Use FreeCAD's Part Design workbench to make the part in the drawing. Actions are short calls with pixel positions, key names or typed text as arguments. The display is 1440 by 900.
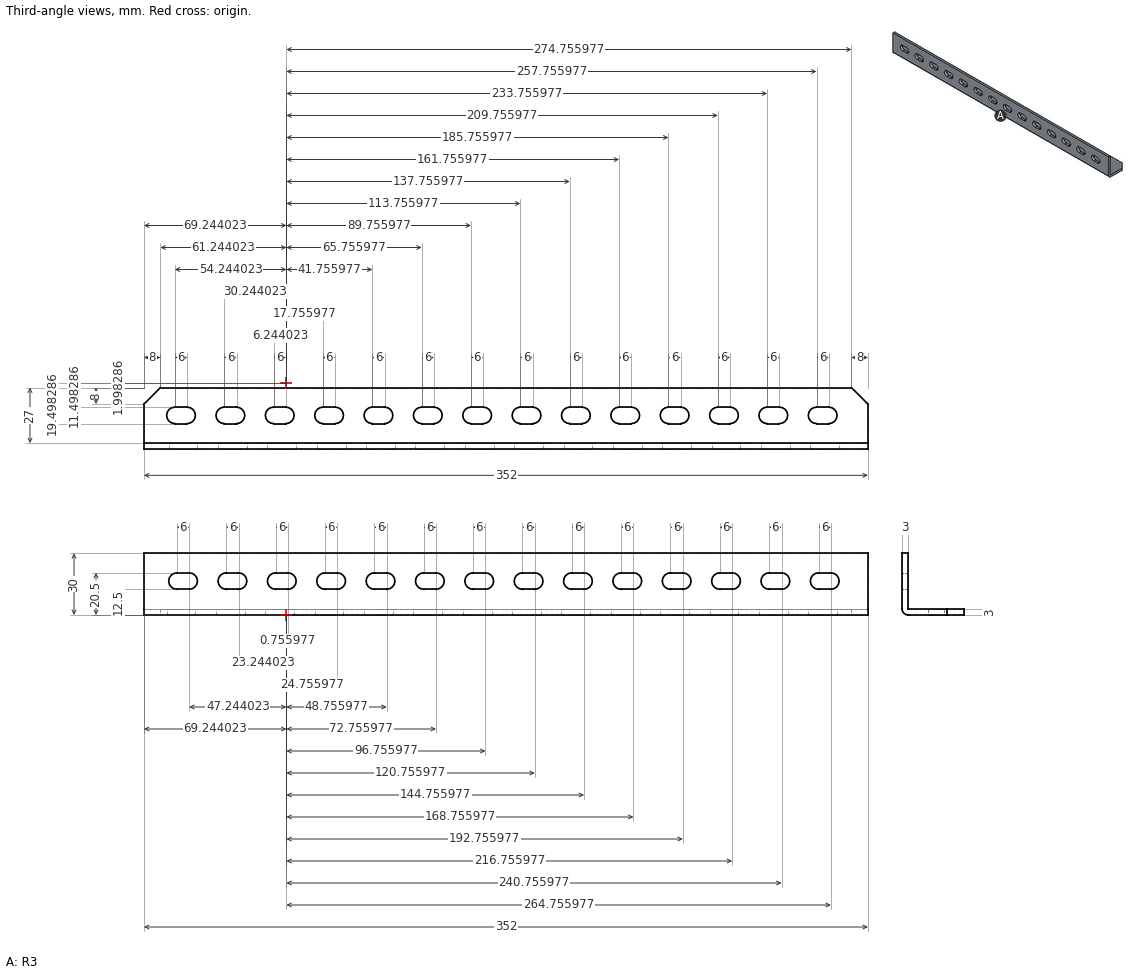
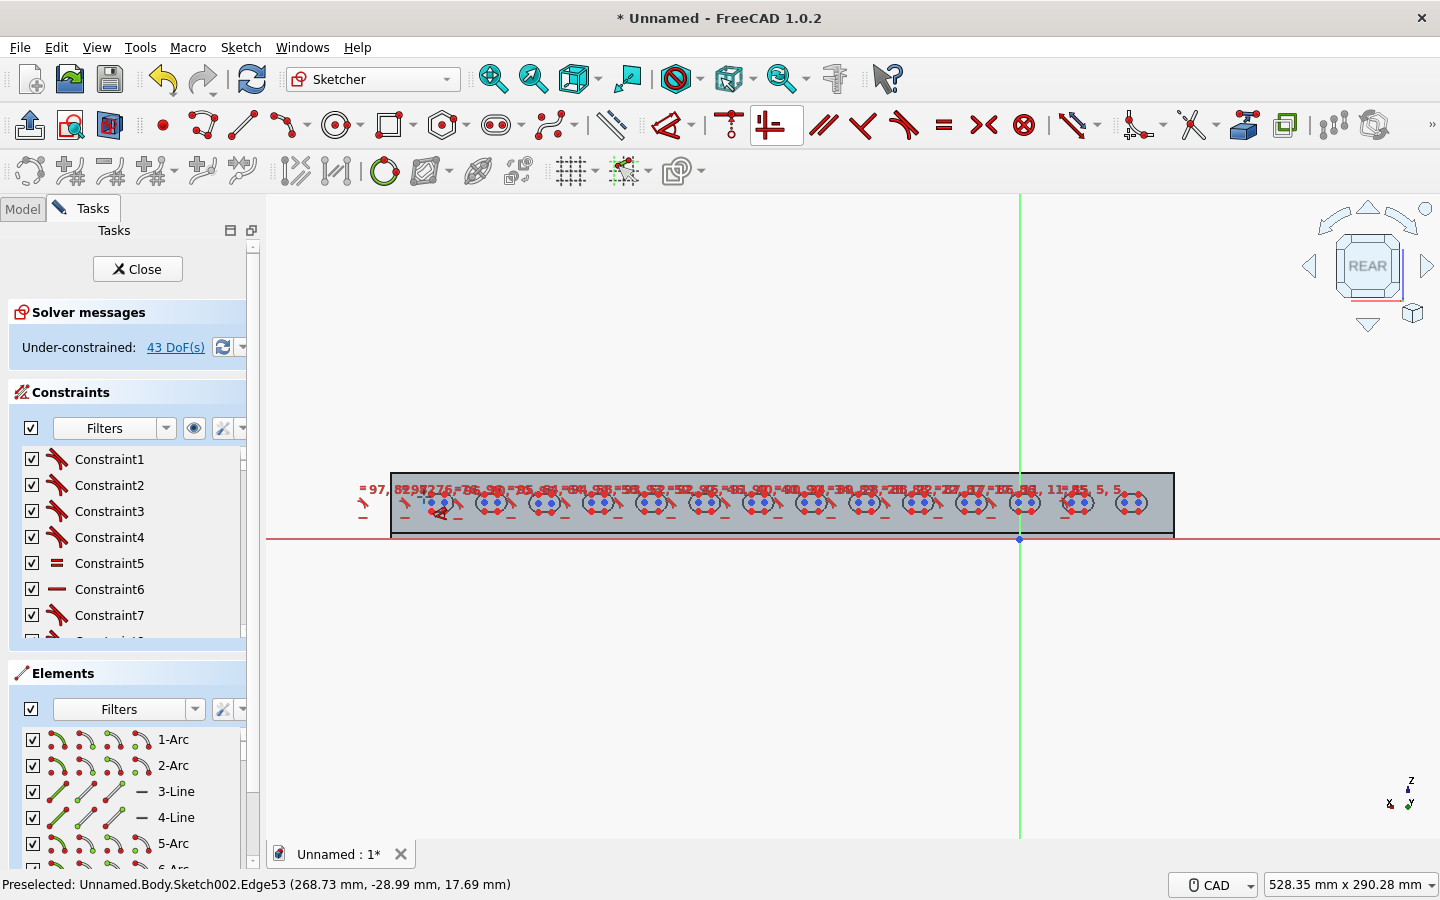
scroll(1130, 494, up, 6)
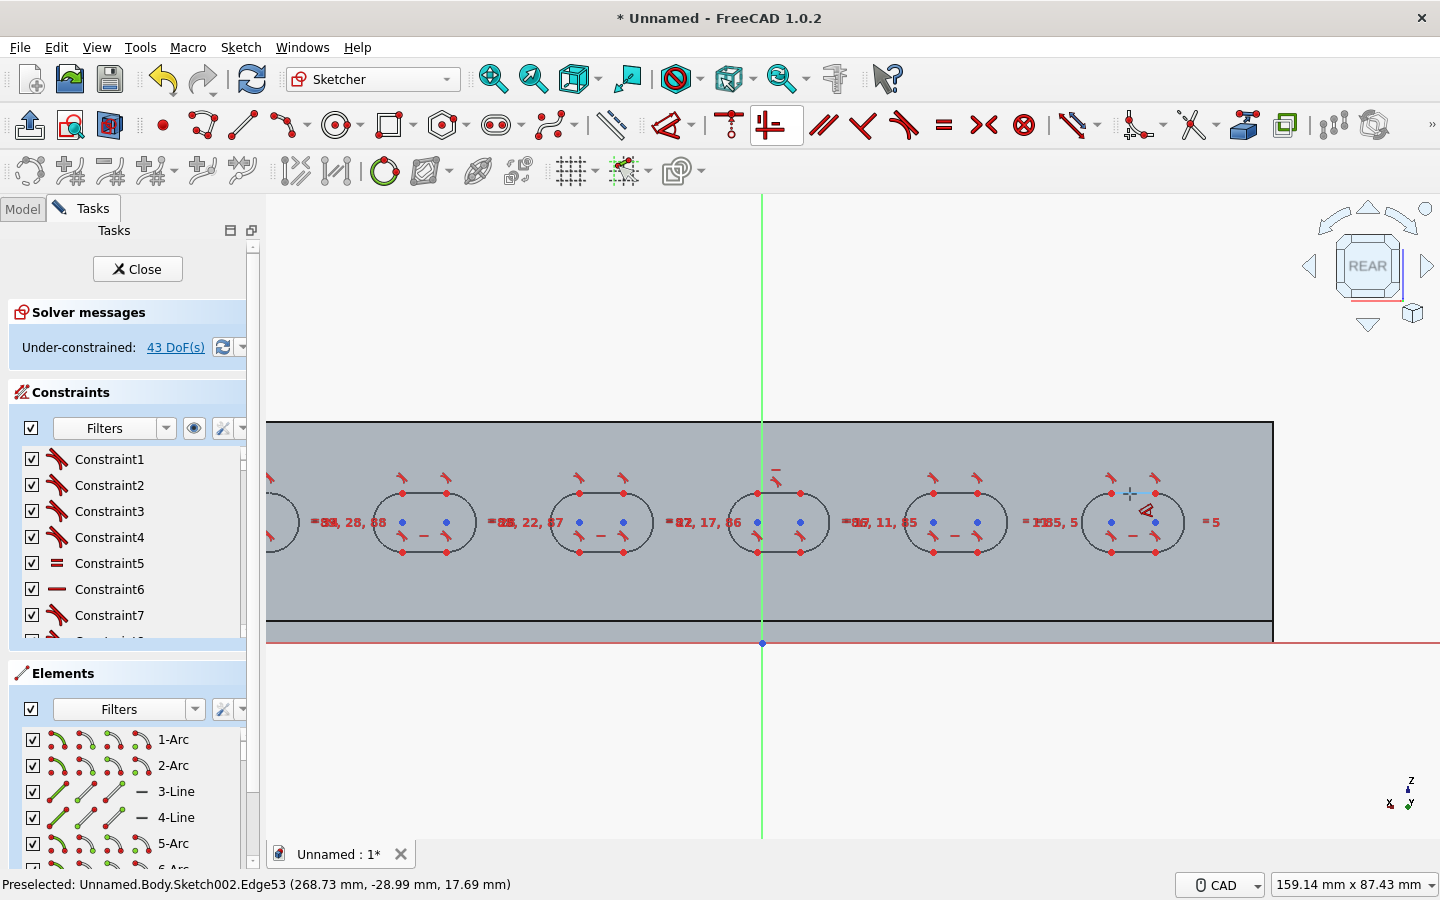
click(1129, 493)
click(1133, 459)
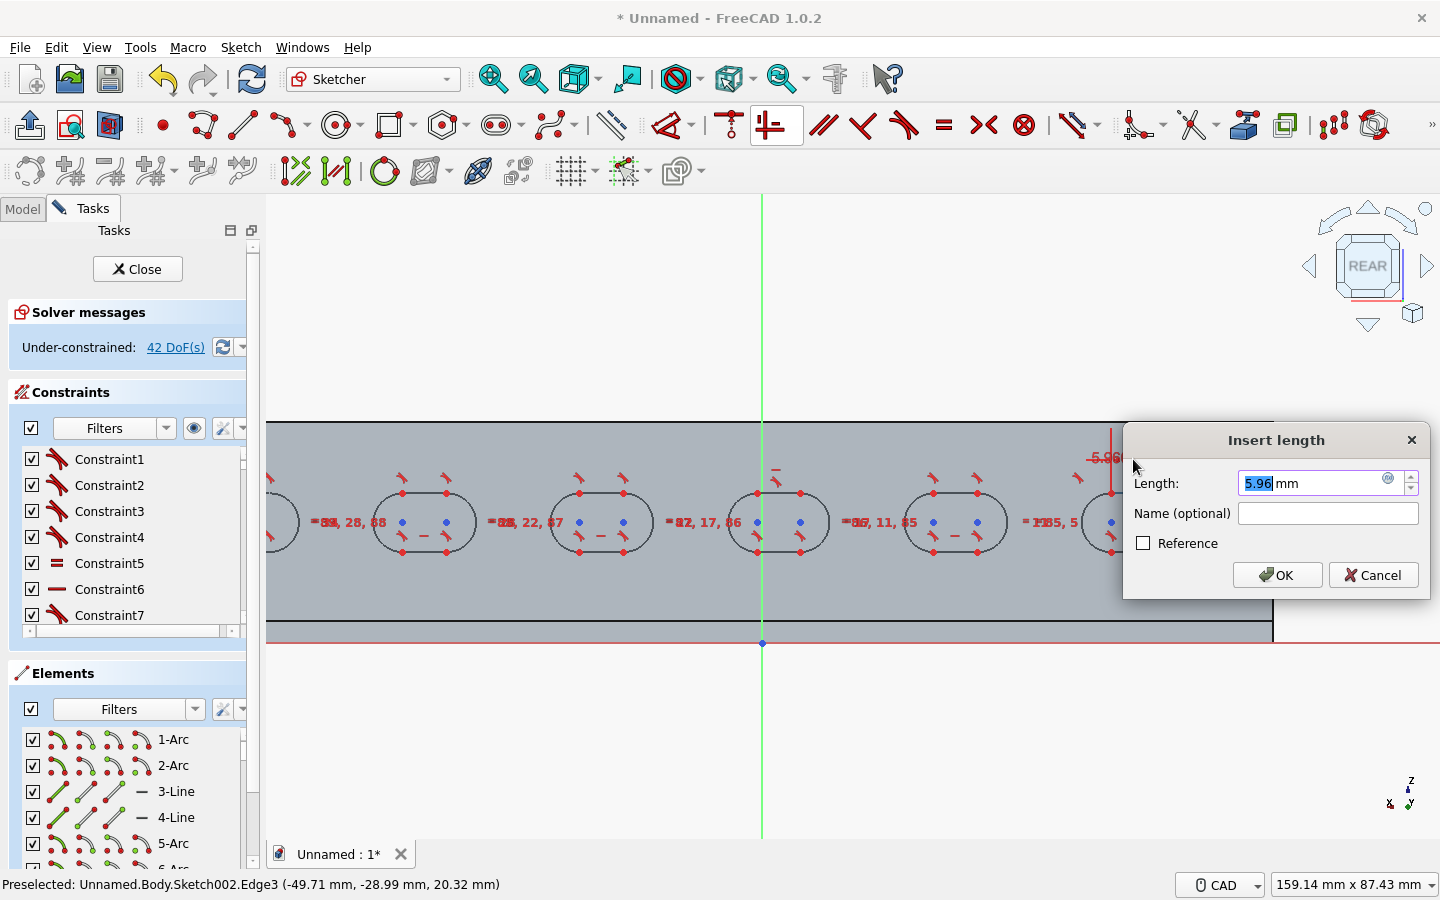
text(6)
key(Return)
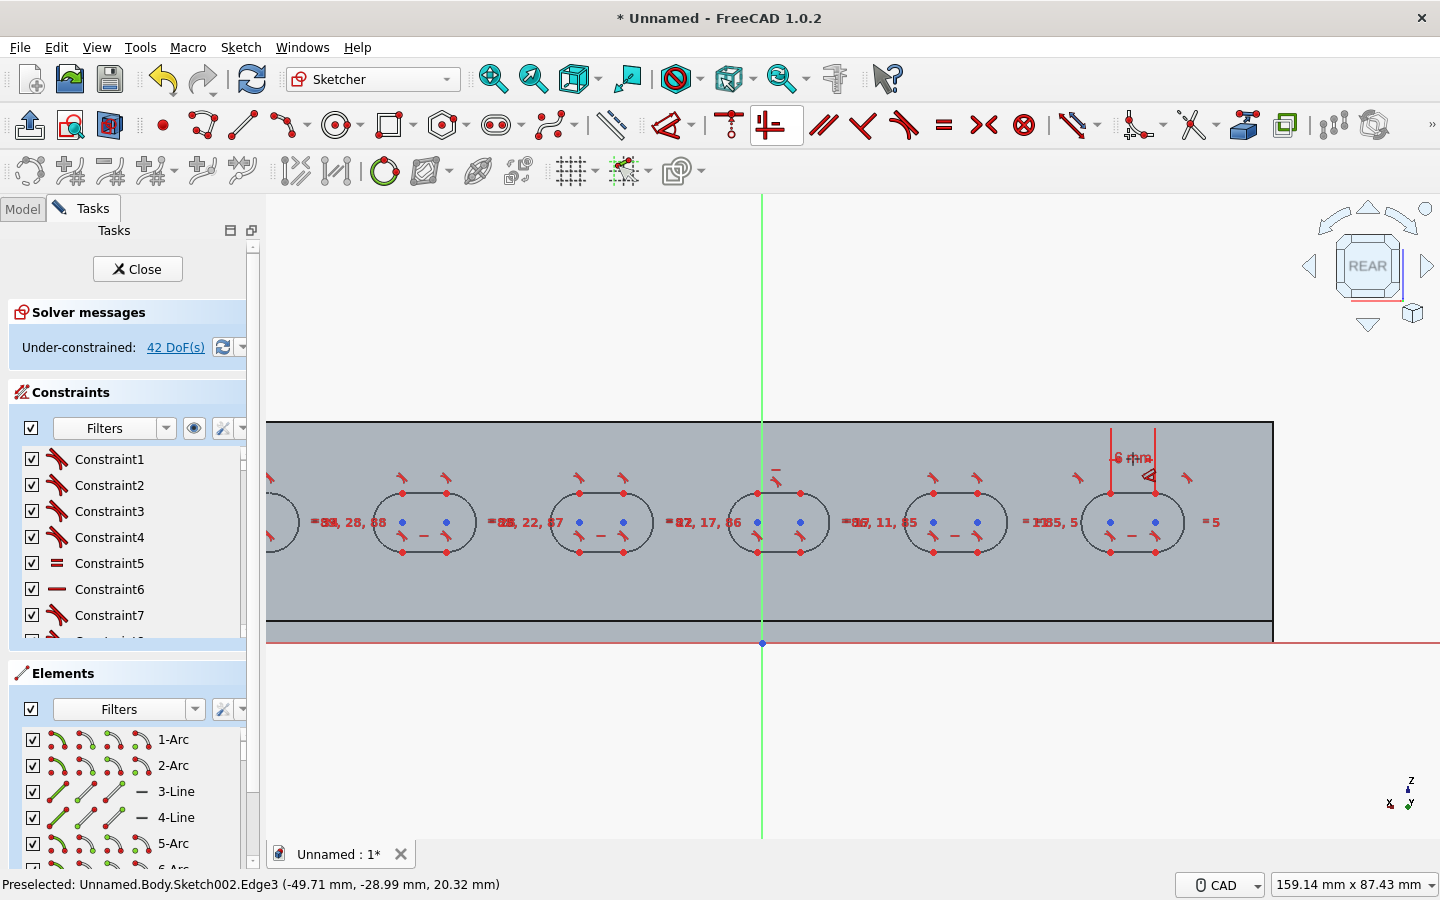
click(947, 493)
click(956, 459)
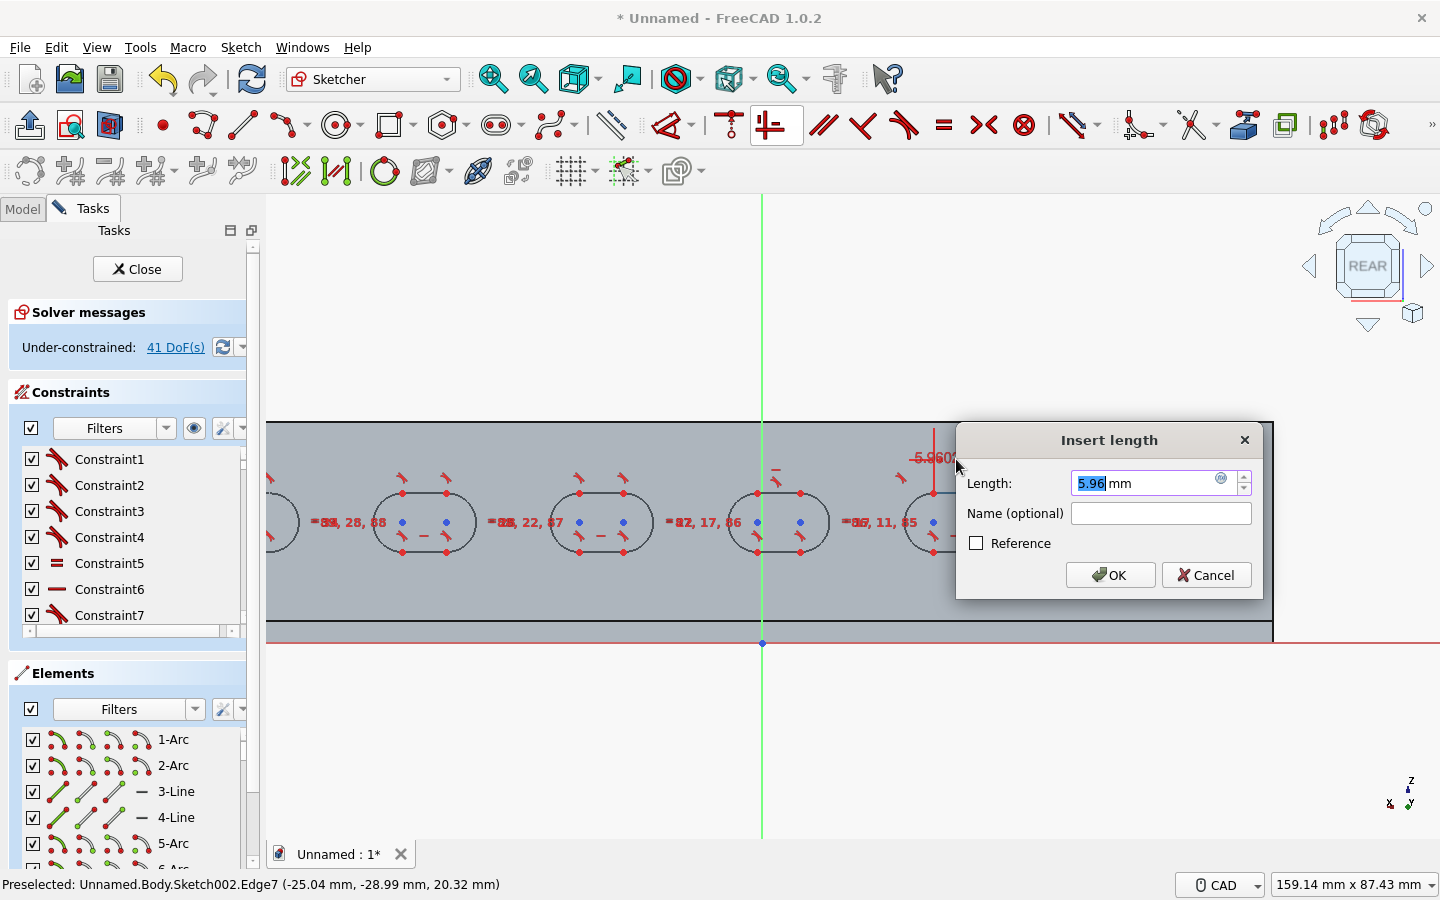
text(6)
key(Return)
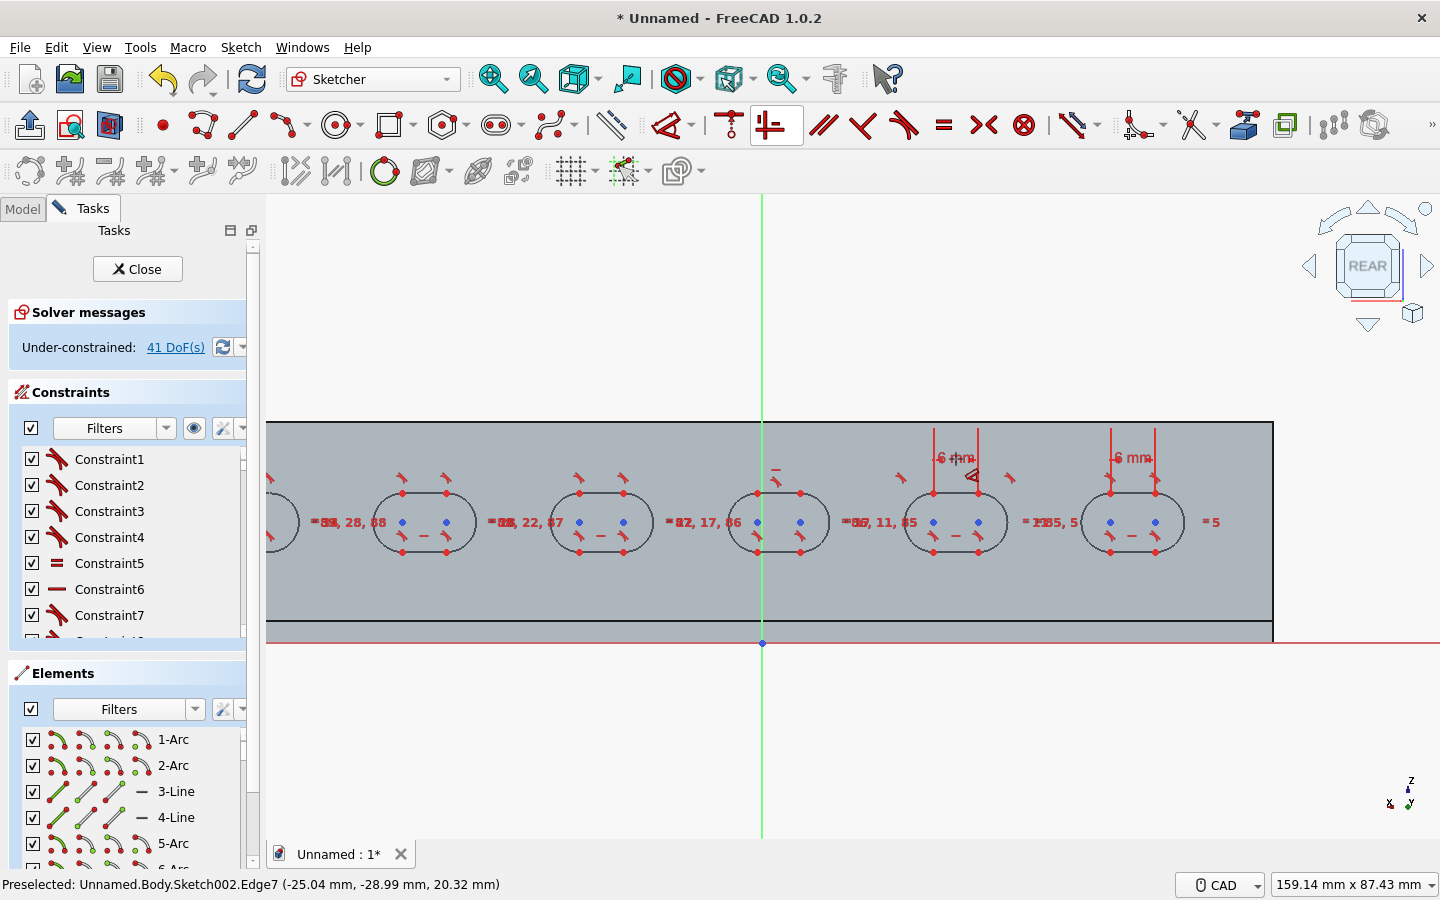
click(787, 493)
click(779, 459)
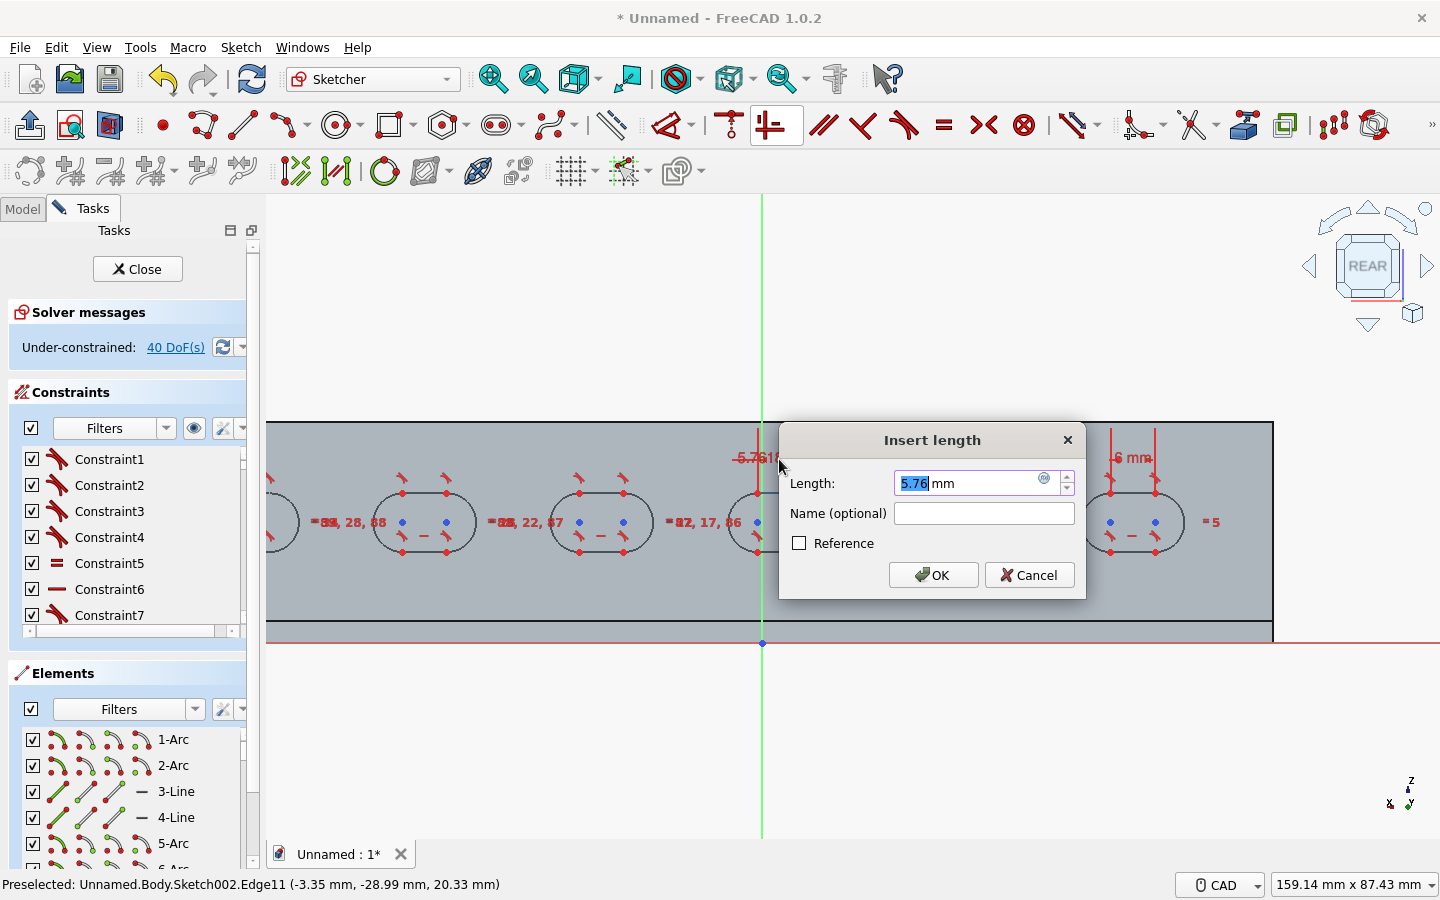
text(6)
key(Return)